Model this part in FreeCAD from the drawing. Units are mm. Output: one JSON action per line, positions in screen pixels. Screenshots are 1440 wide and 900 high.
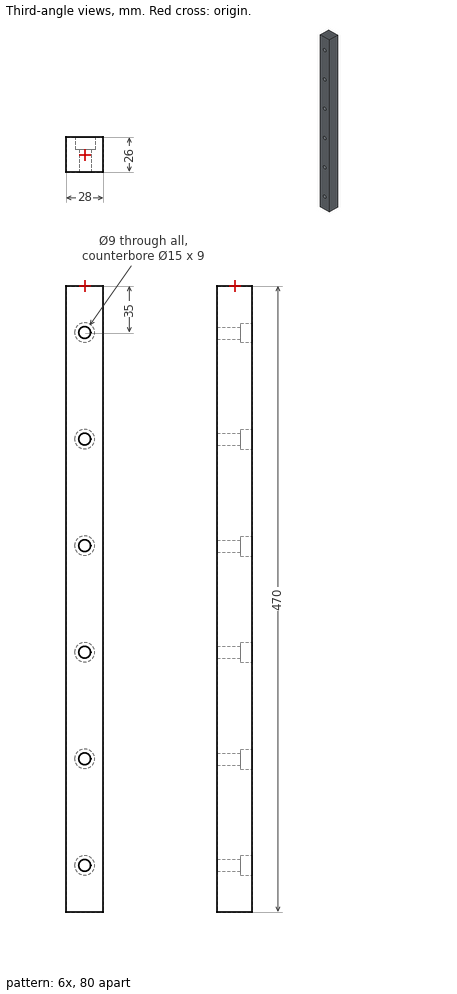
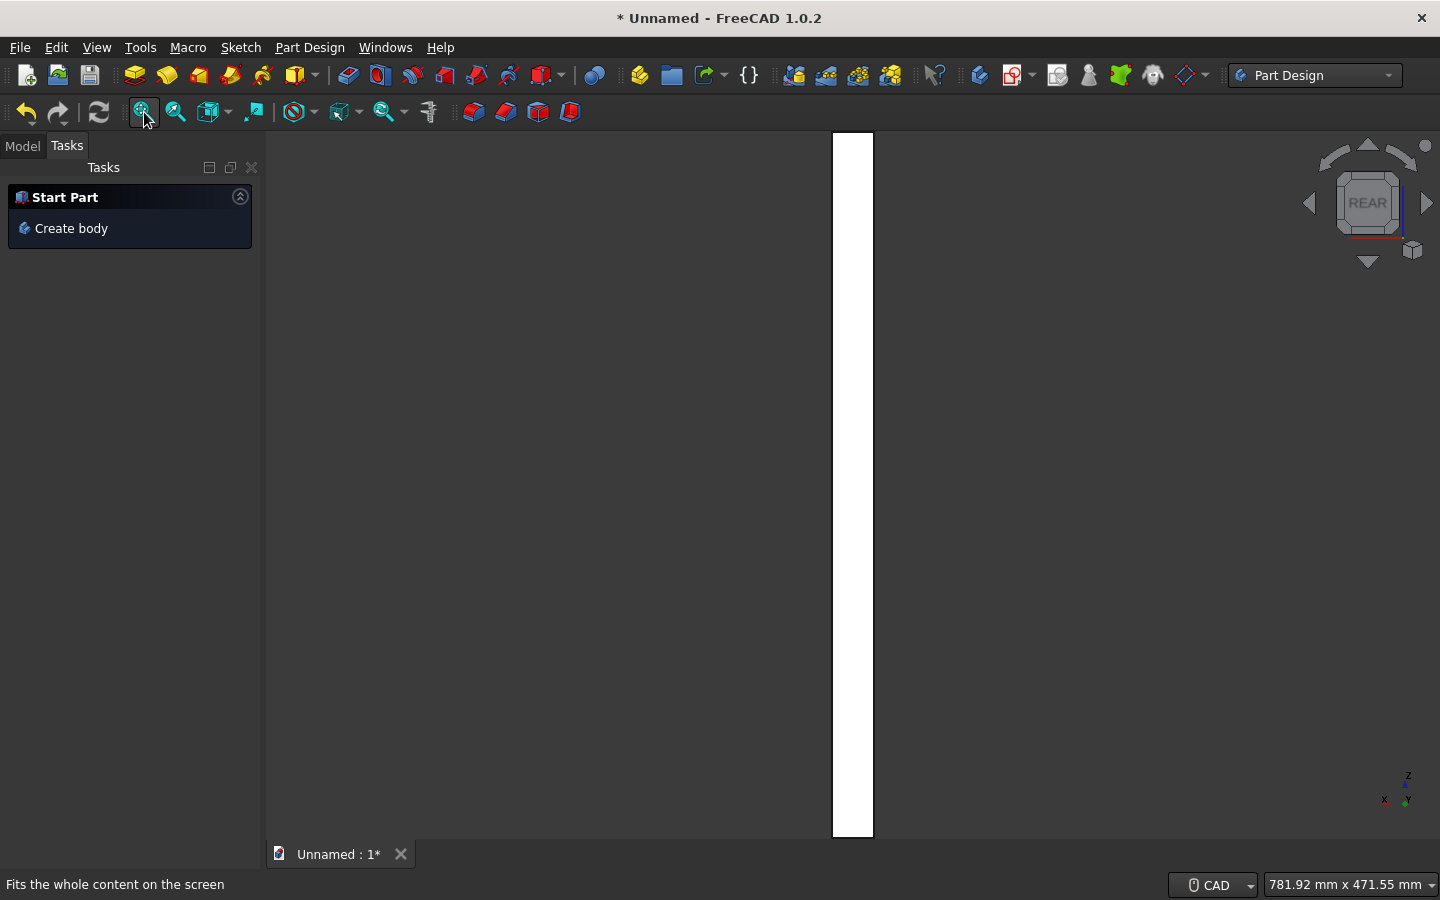
{"action": "left_click", "coordinate": [853, 182]}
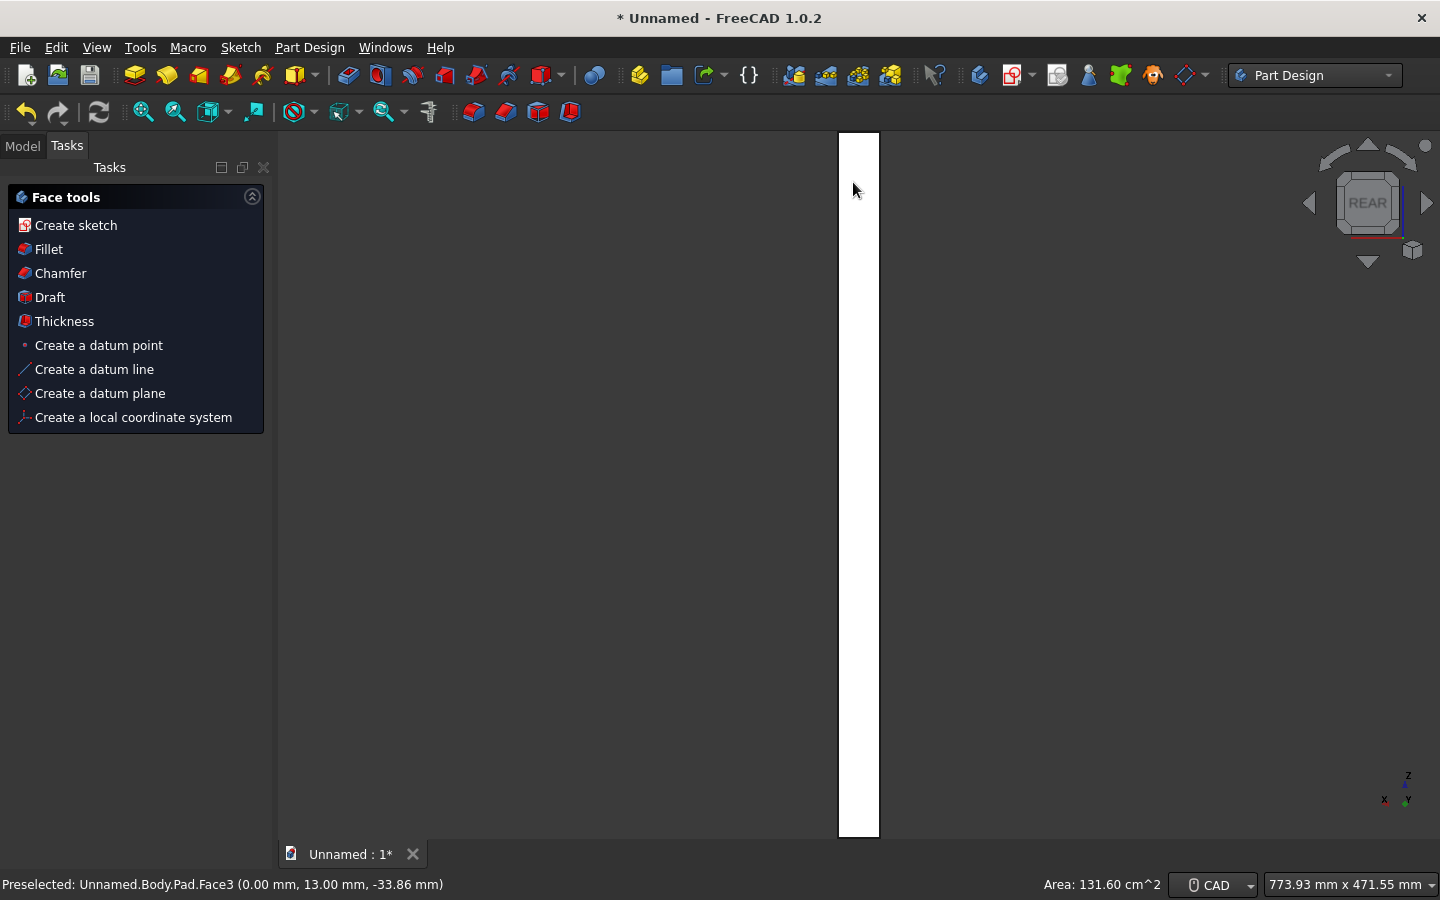
{"action": "left_click", "coordinate": [1012, 76]}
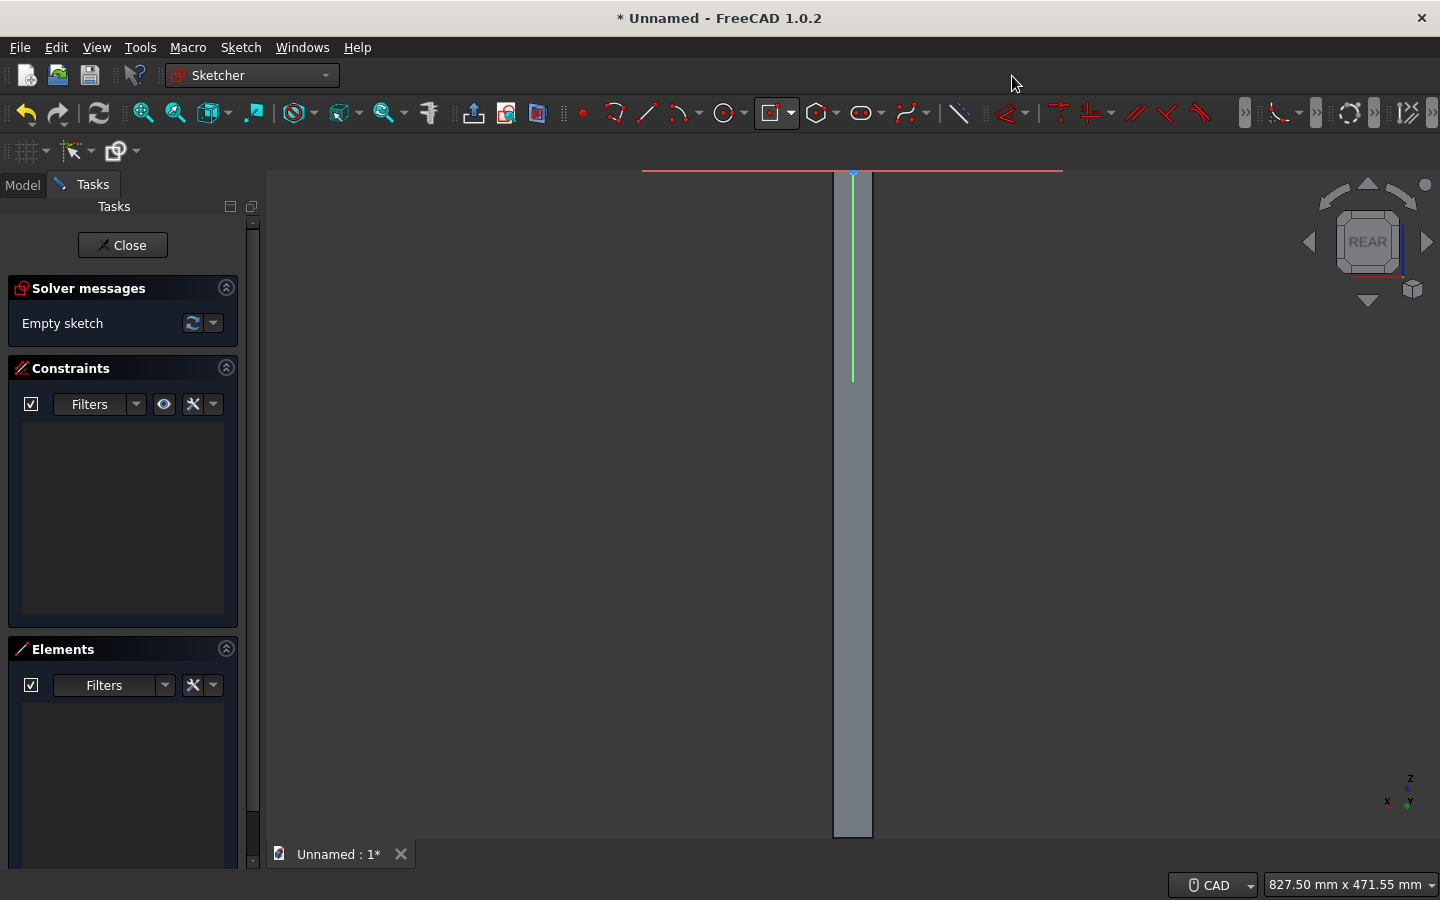
{"action": "scroll", "coordinate": [857, 206], "scroll_direction": "up", "scroll_amount": 15}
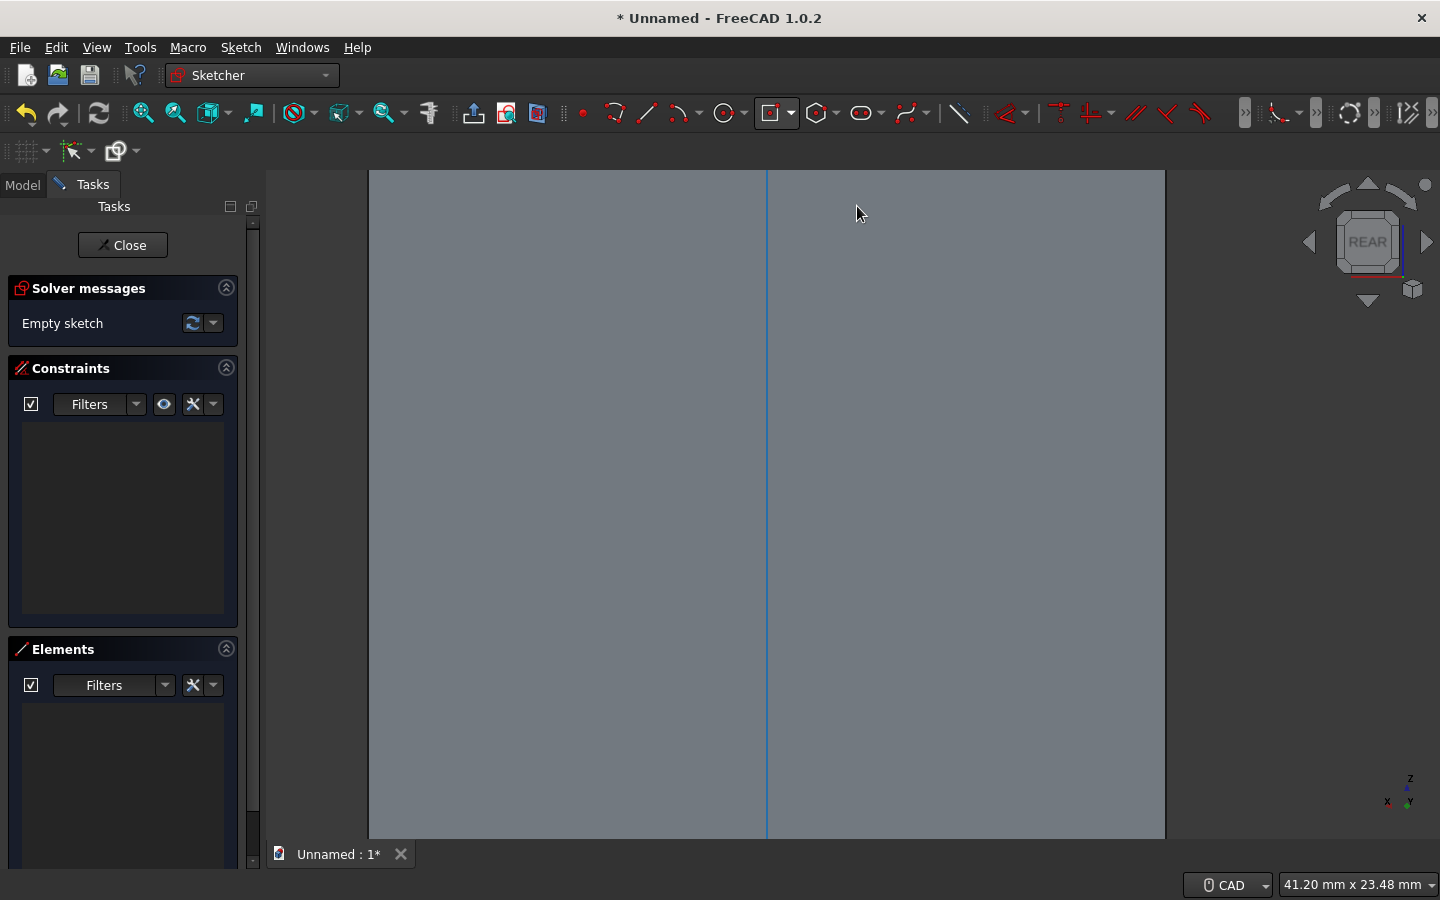
{"action": "scroll", "coordinate": [746, 497], "scroll_direction": "up", "scroll_amount": 3}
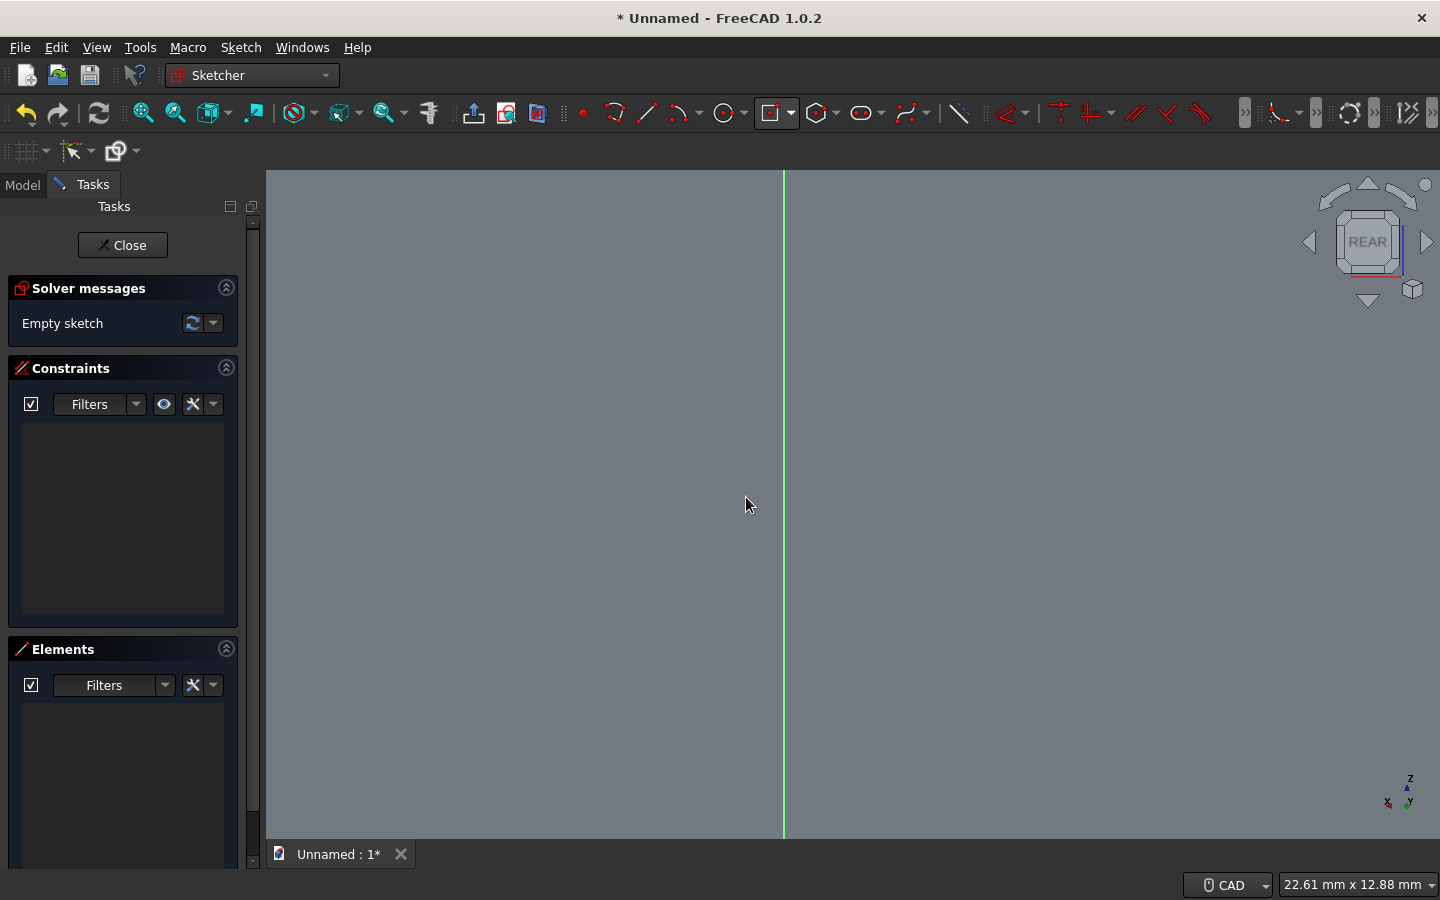
{"action": "left_click", "coordinate": [724, 114]}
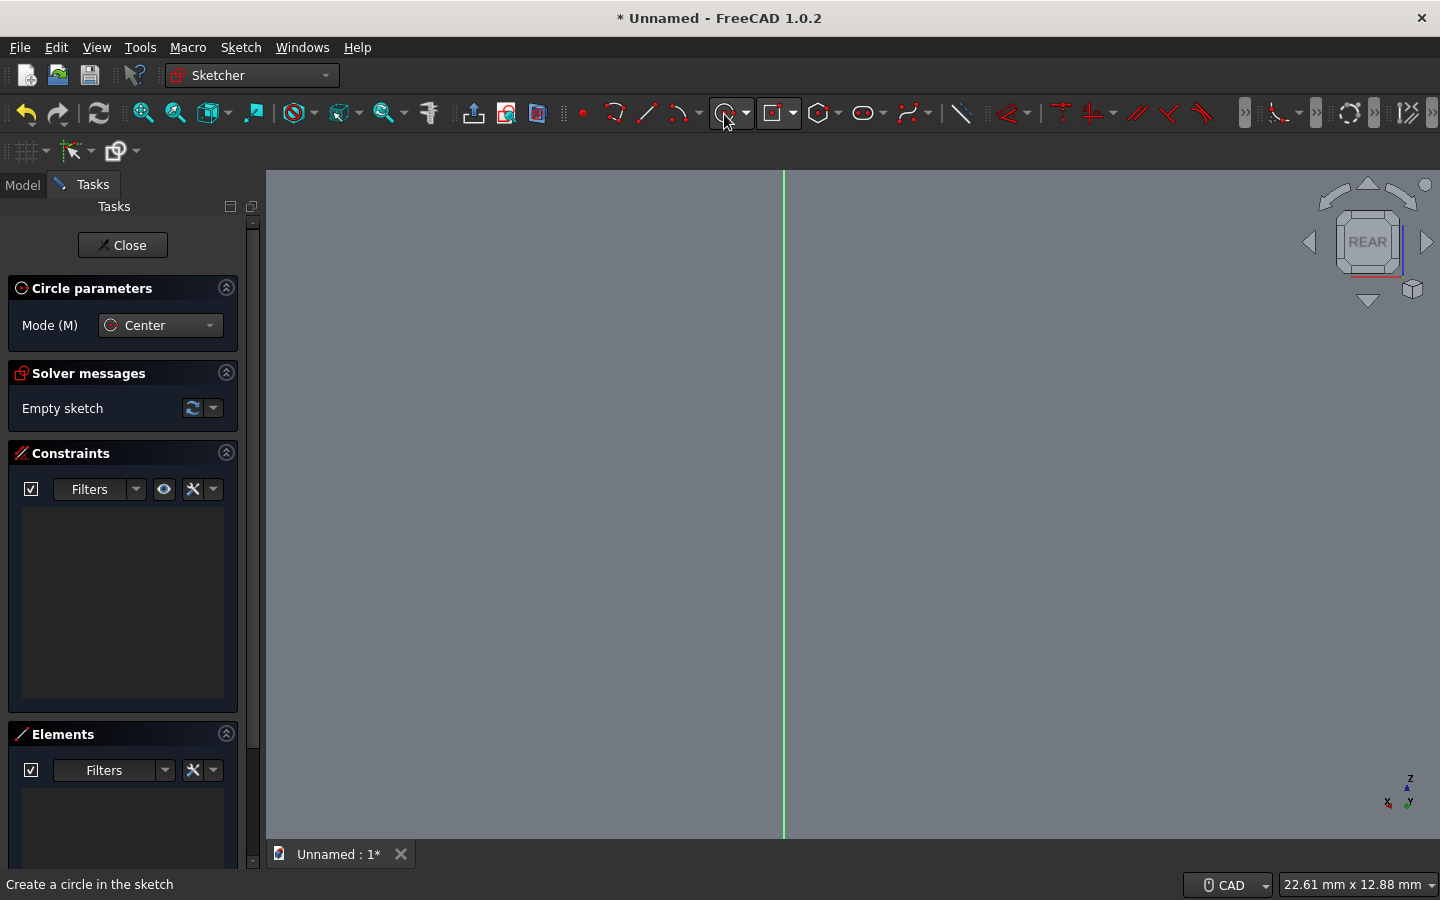
{"action": "left_click", "coordinate": [784, 505]}
{"action": "mouse_move", "coordinate": [949, 339]}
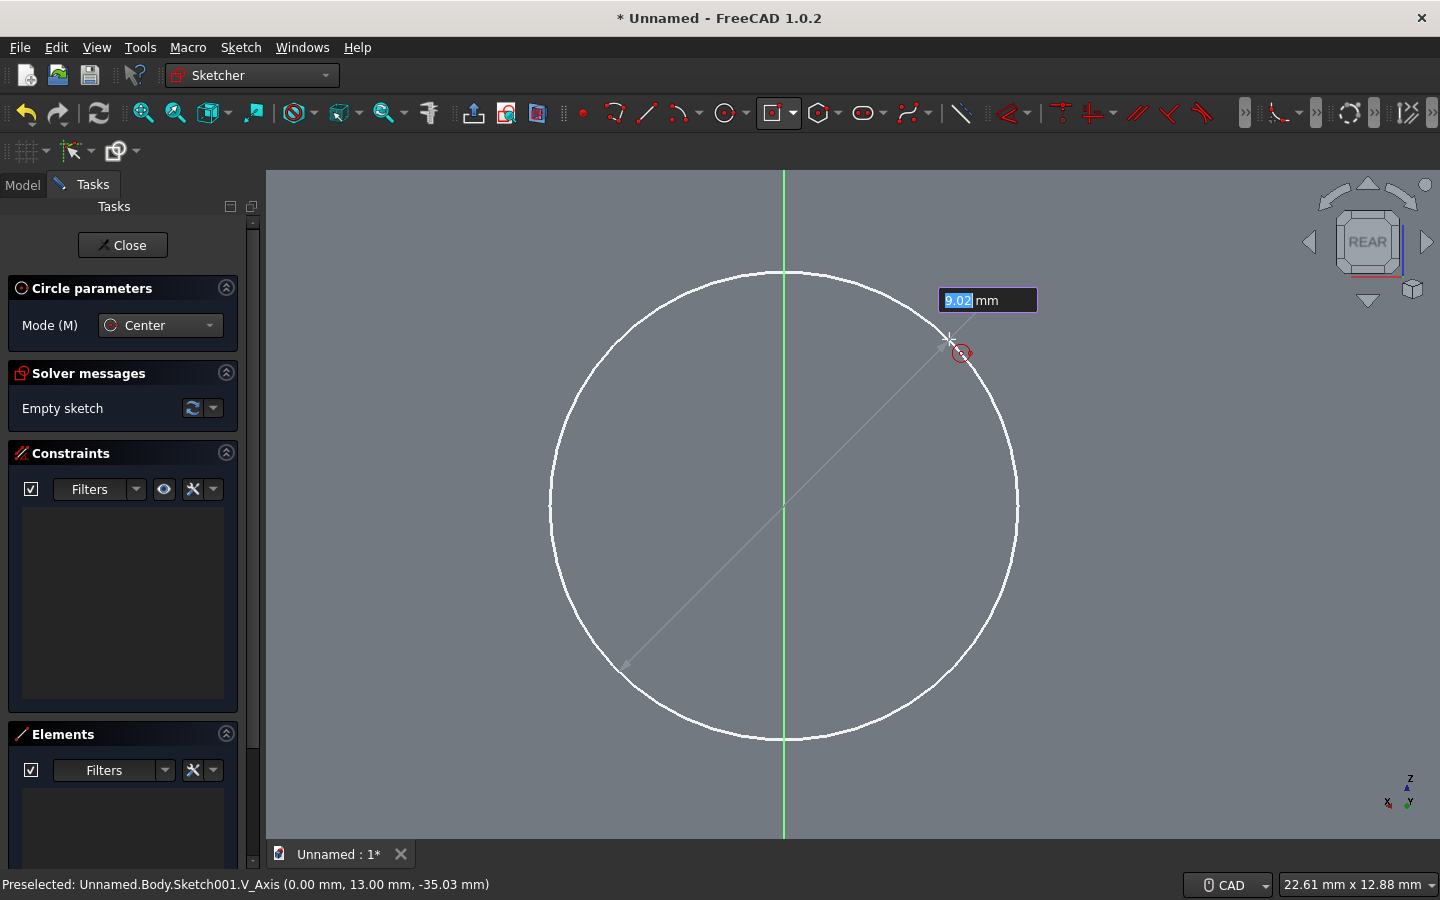
{"action": "type", "text": "9"}
{"action": "key", "text": "Return"}
{"action": "key", "text": "Escape"}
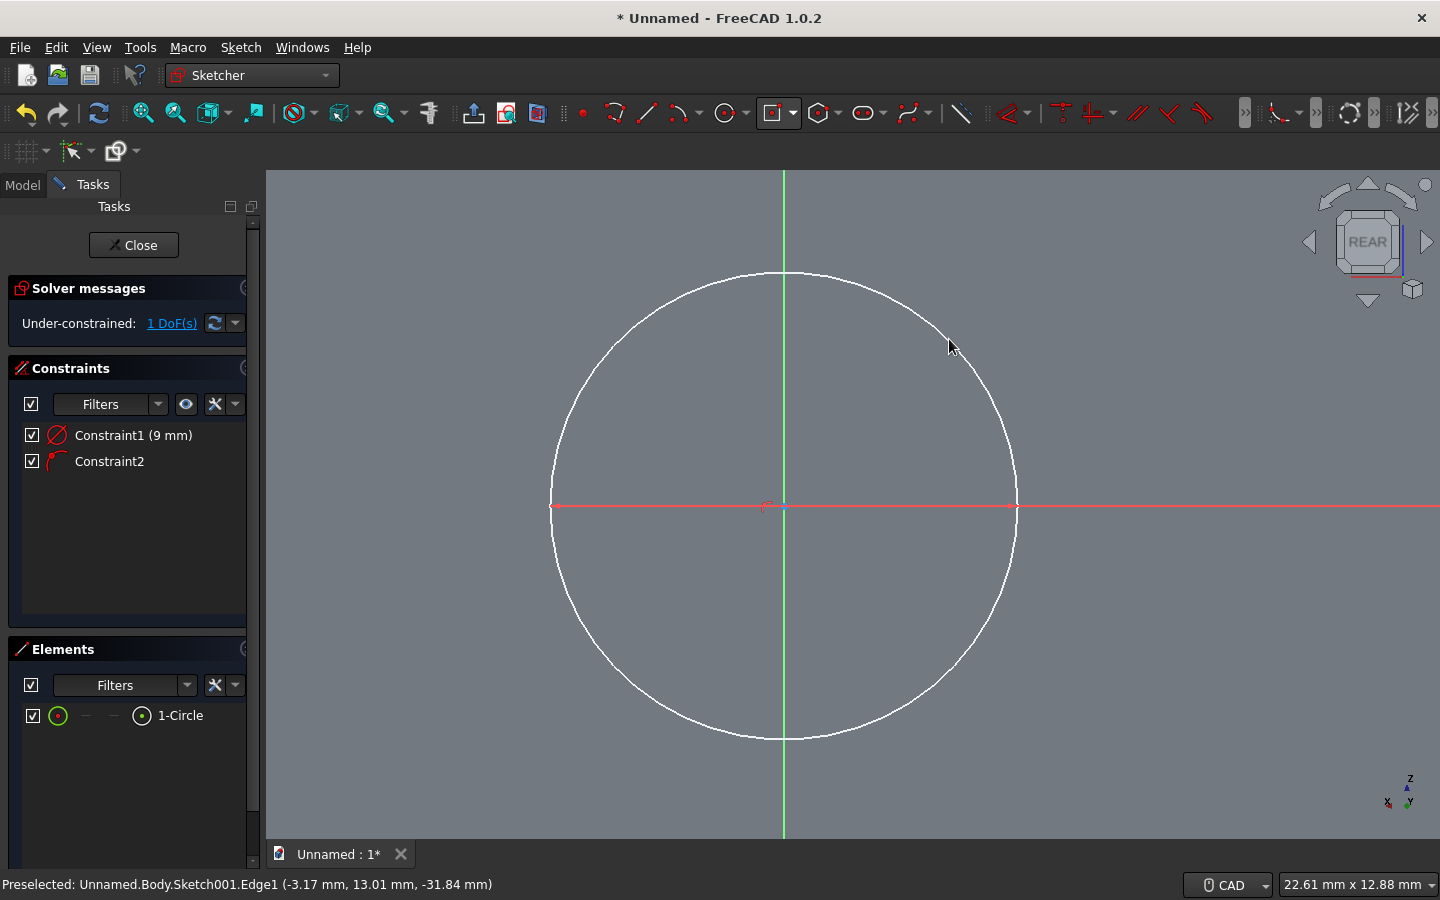
{"action": "left_click", "coordinate": [1008, 114]}